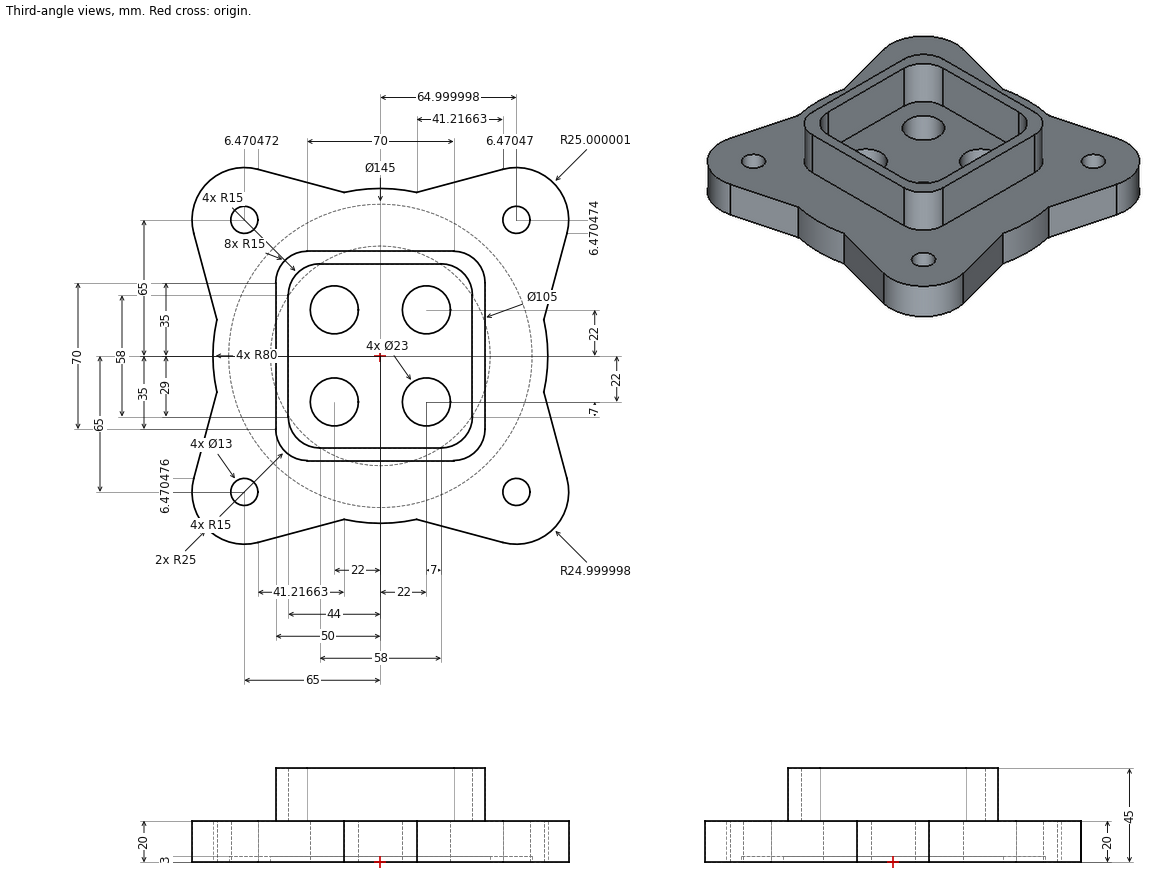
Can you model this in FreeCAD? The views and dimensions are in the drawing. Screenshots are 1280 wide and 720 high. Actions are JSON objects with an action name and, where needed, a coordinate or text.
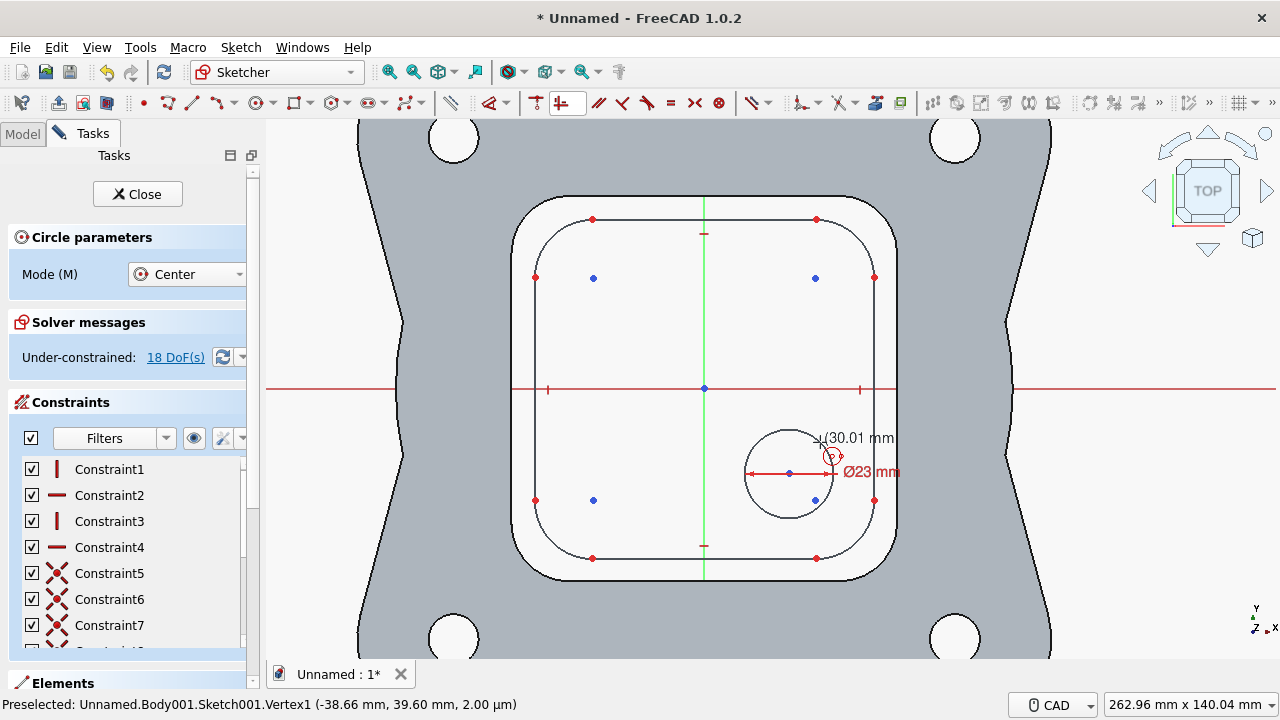
{"action": "left_click", "coordinate": [619, 473]}
{"action": "mouse_move", "coordinate": [651, 442]}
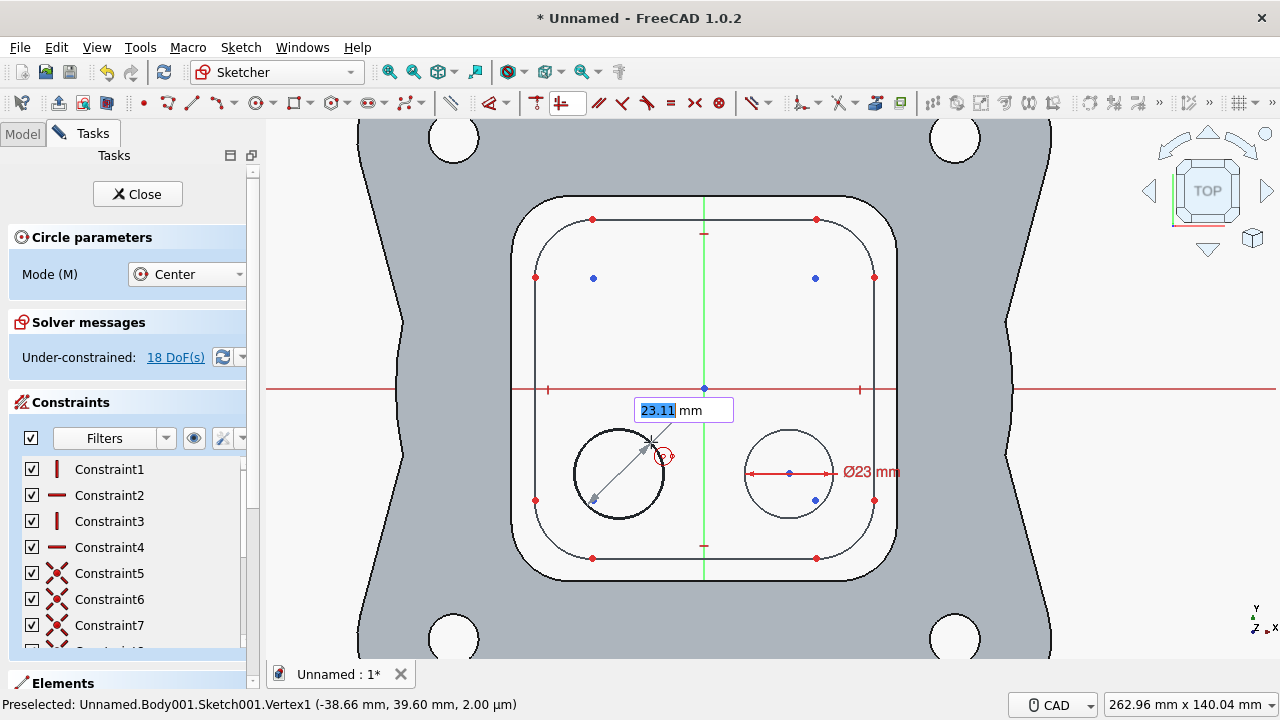
{"action": "type", "text": "23"}
{"action": "key", "text": "Return"}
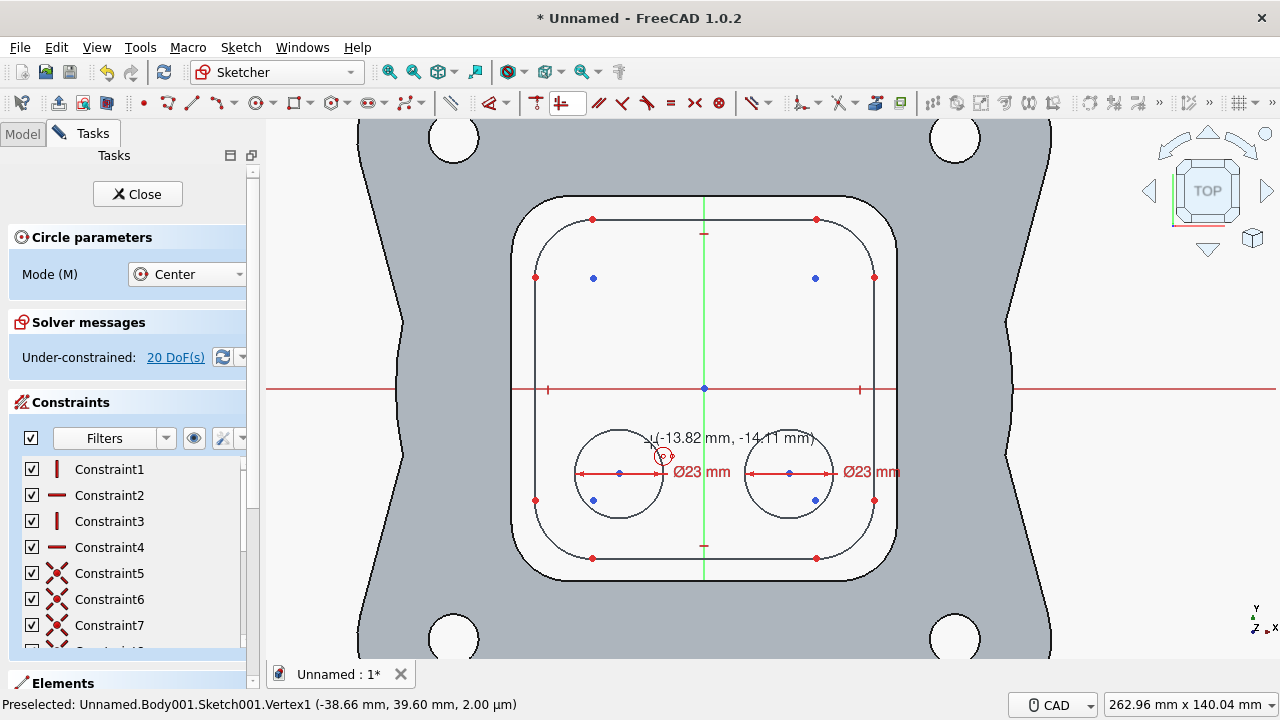
{"action": "left_click", "coordinate": [789, 304]}
{"action": "mouse_move", "coordinate": [758, 272]}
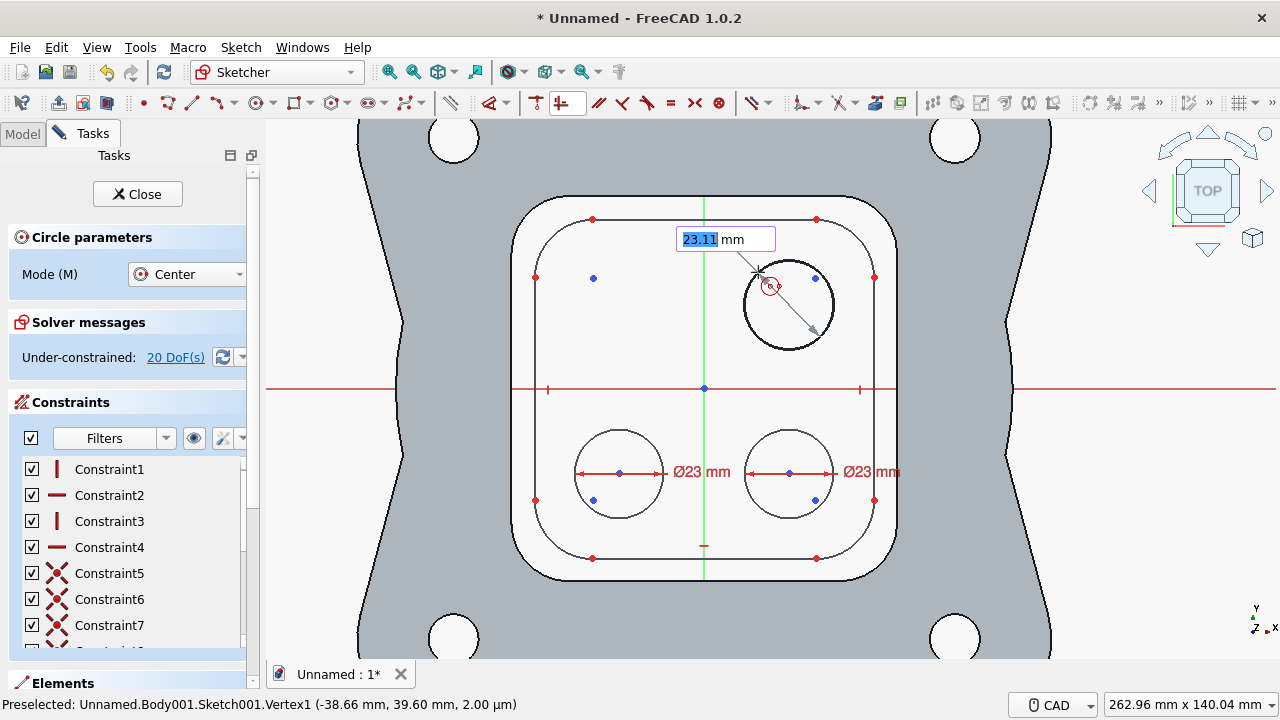
{"action": "type", "text": "23"}
{"action": "key", "text": "Return"}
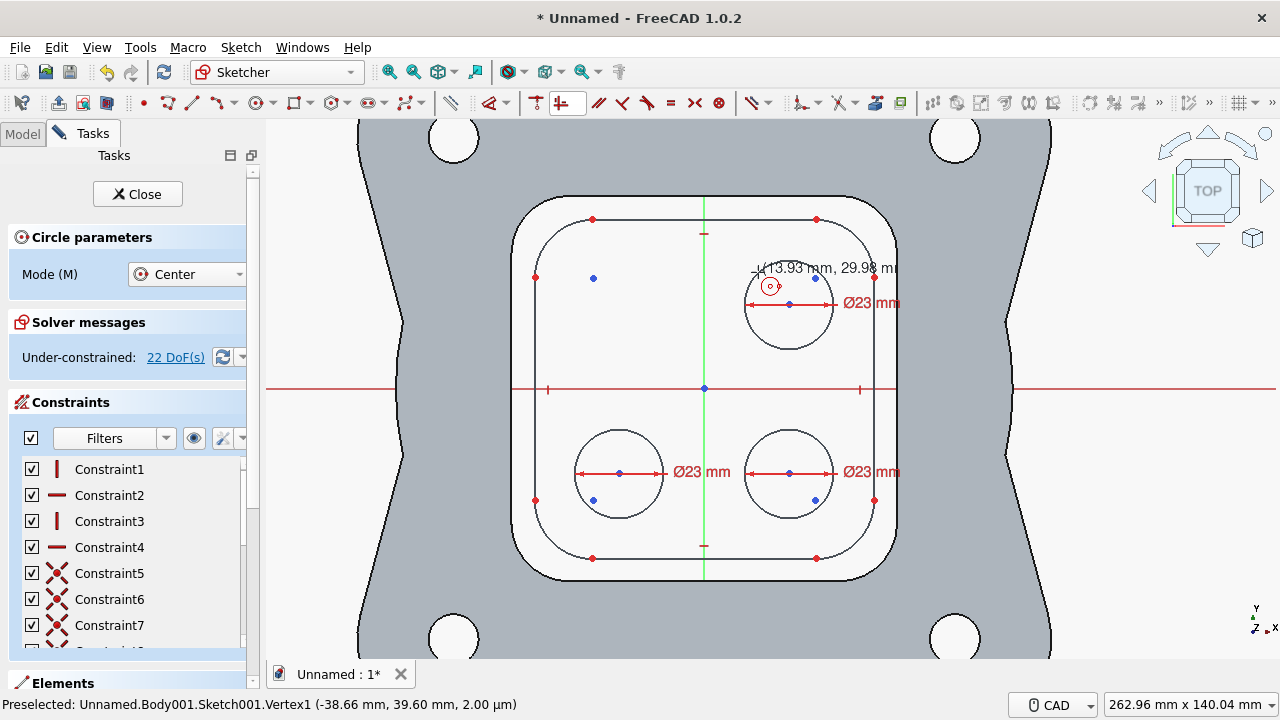
{"action": "left_click", "coordinate": [619, 304]}
{"action": "mouse_move", "coordinate": [651, 272]}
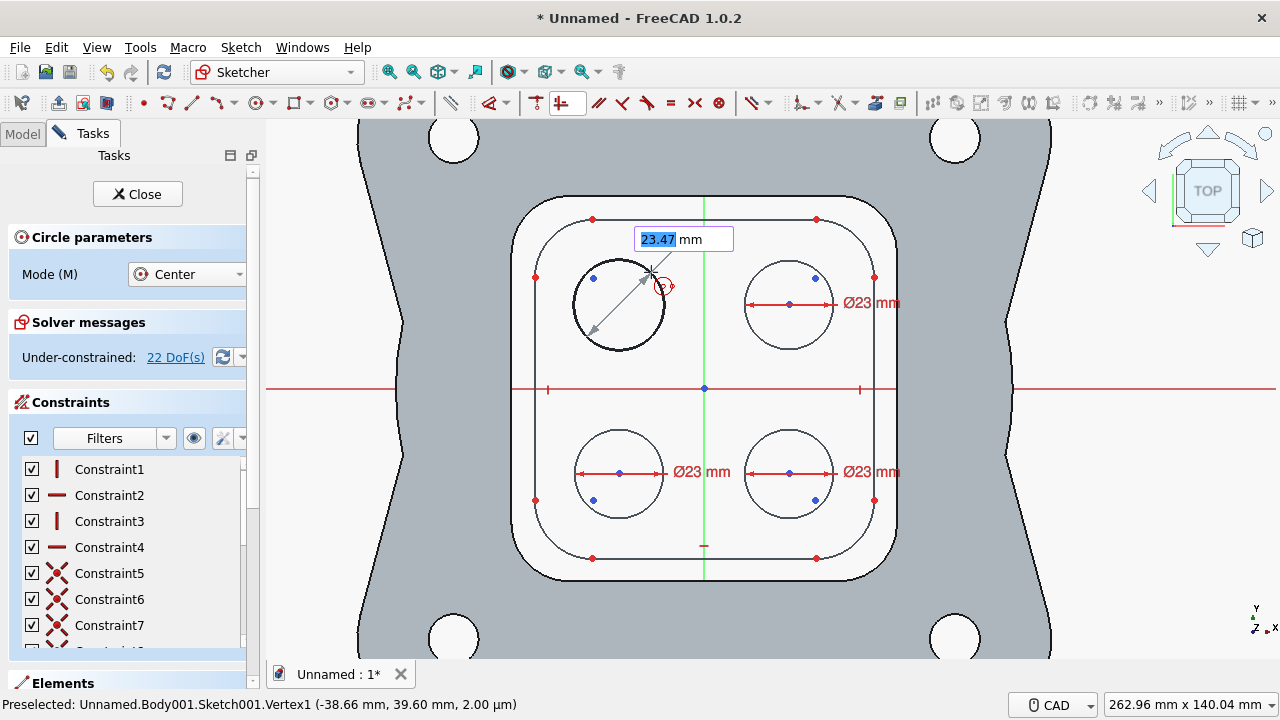
{"action": "type", "text": "23"}
{"action": "key", "text": "Return"}
{"action": "key", "text": "Escape"}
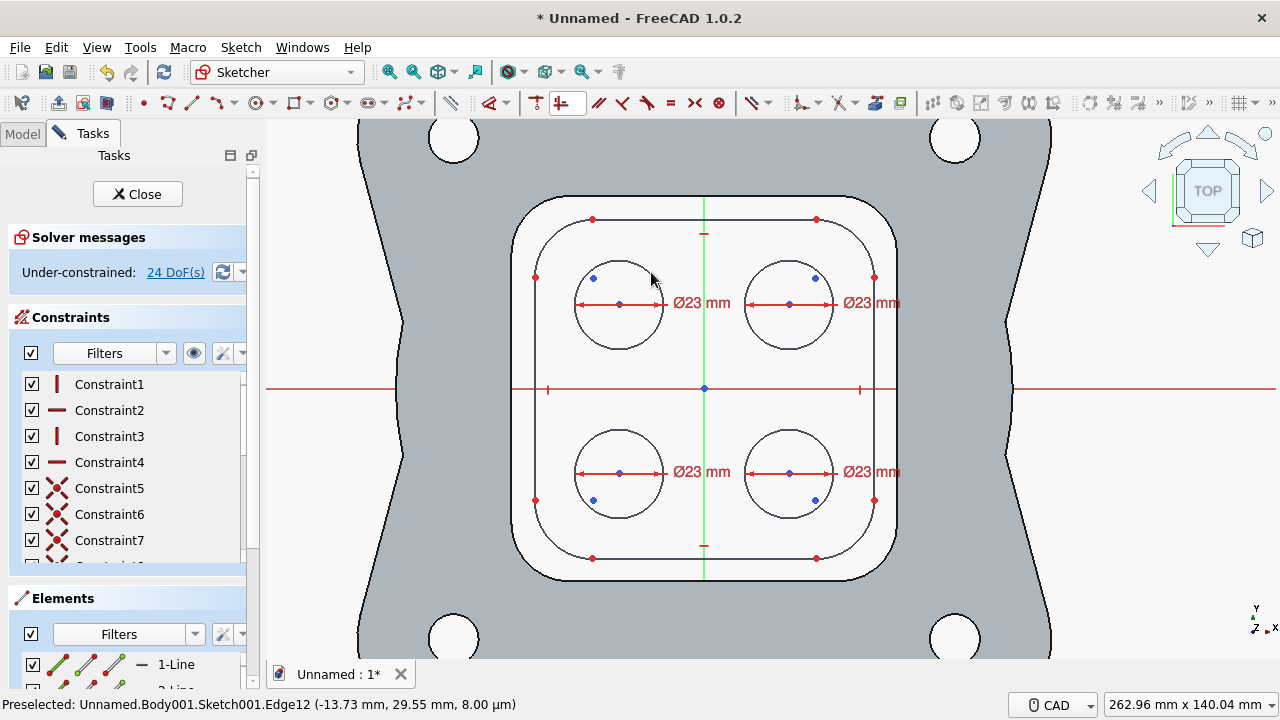
{"action": "left_click", "coordinate": [535, 345]}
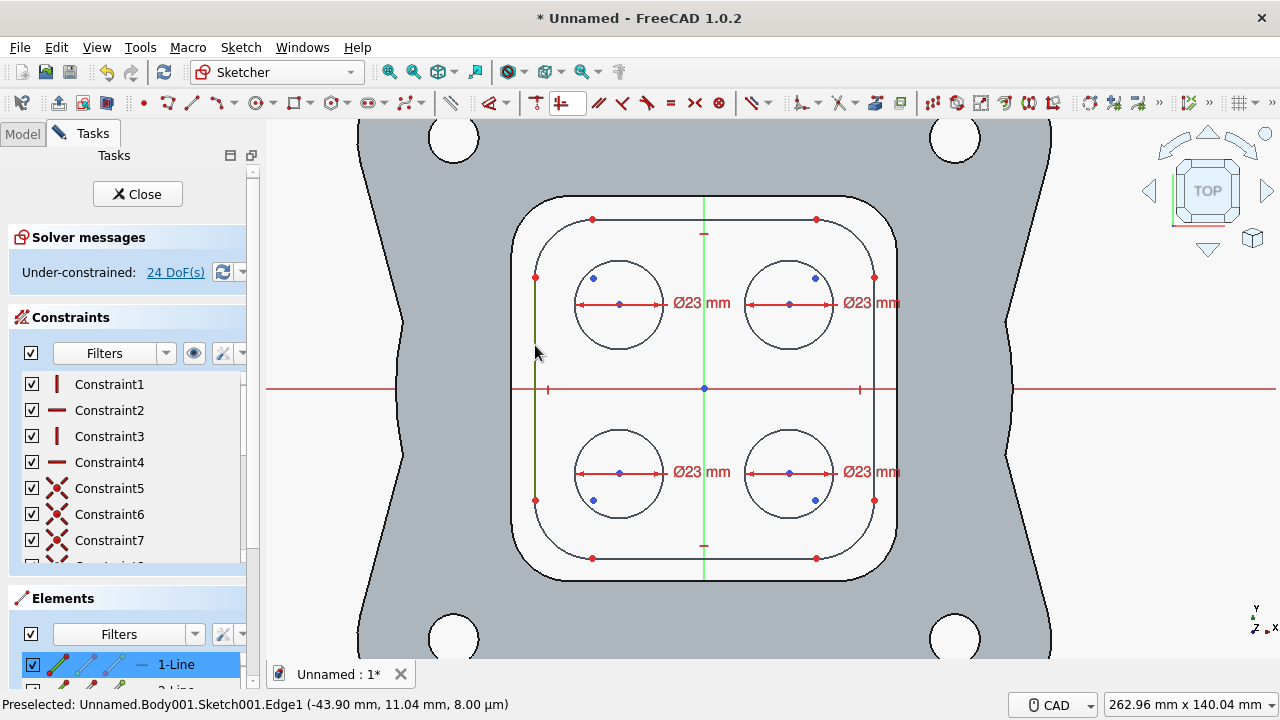
{"action": "left_click", "coordinate": [541, 527]}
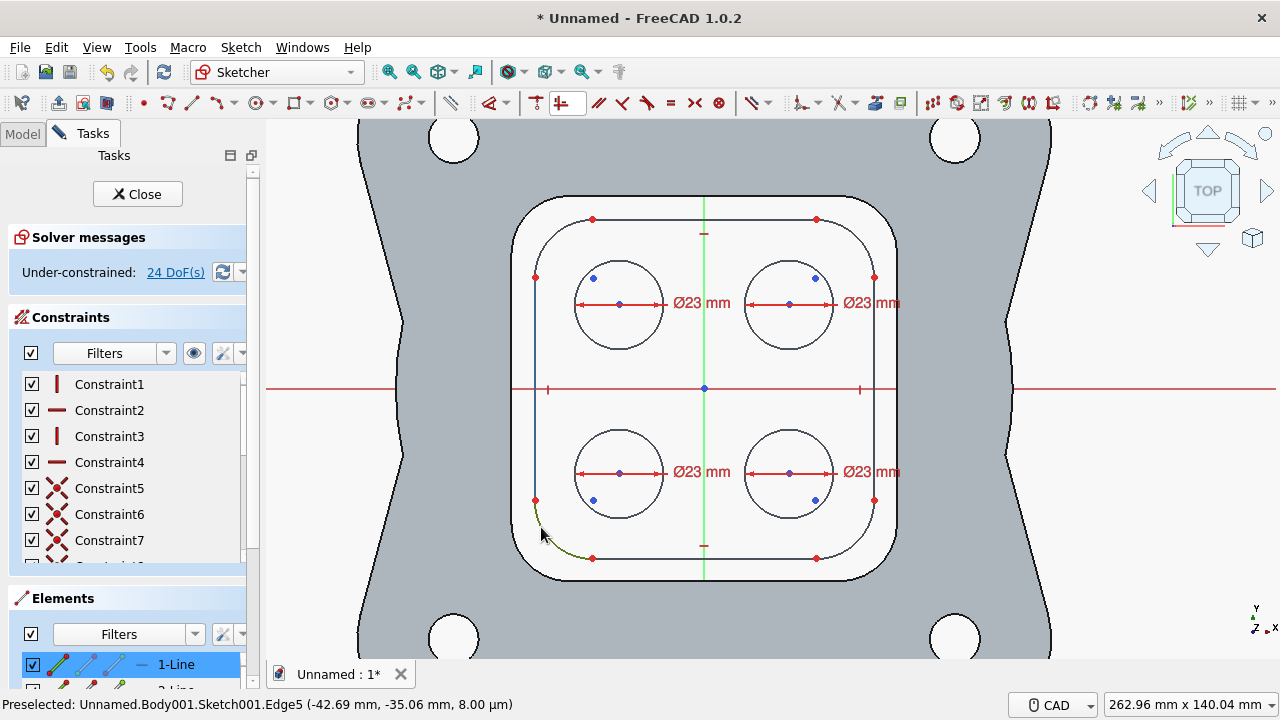
{"action": "left_click", "coordinate": [648, 104]}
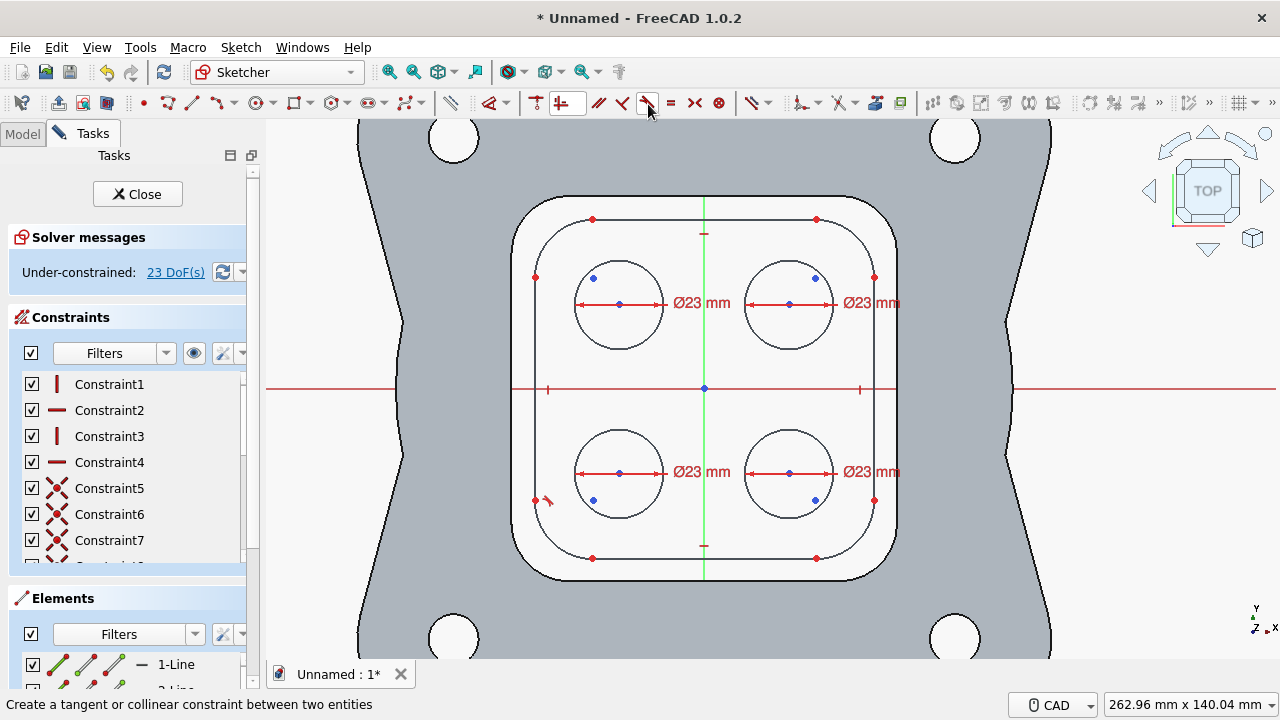
{"action": "left_click", "coordinate": [535, 345]}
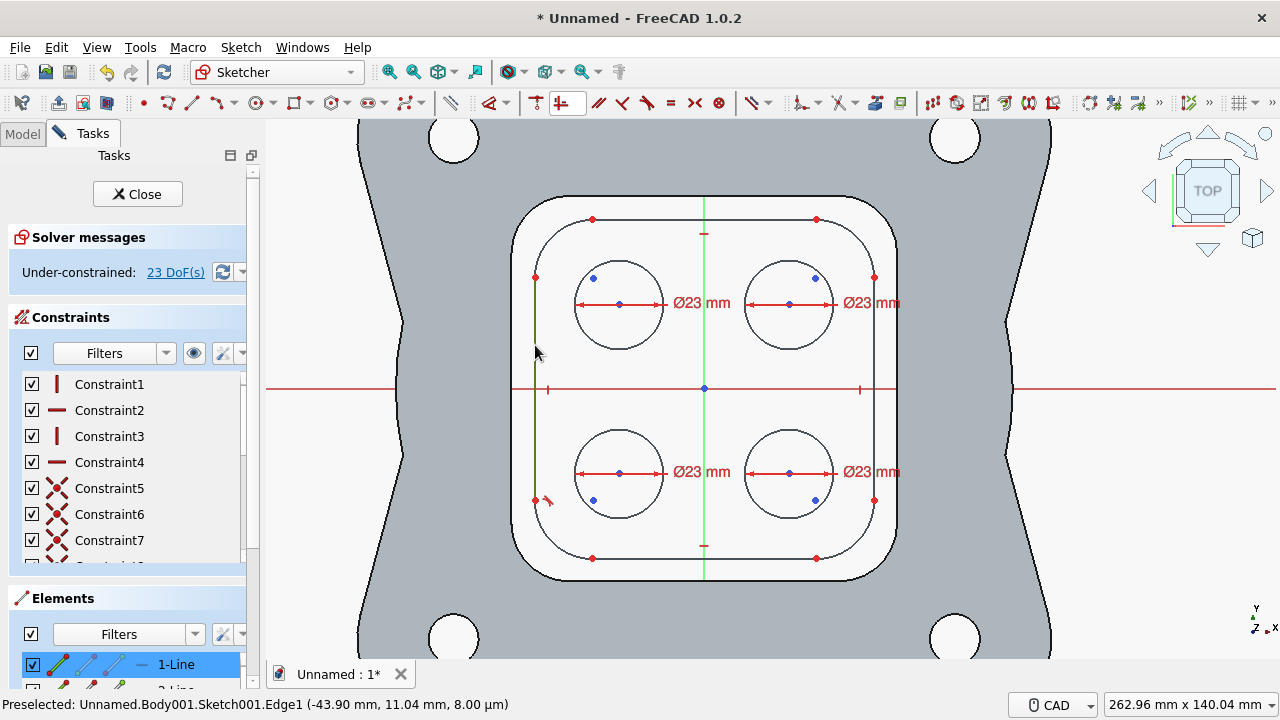
{"action": "left_click", "coordinate": [566, 227]}